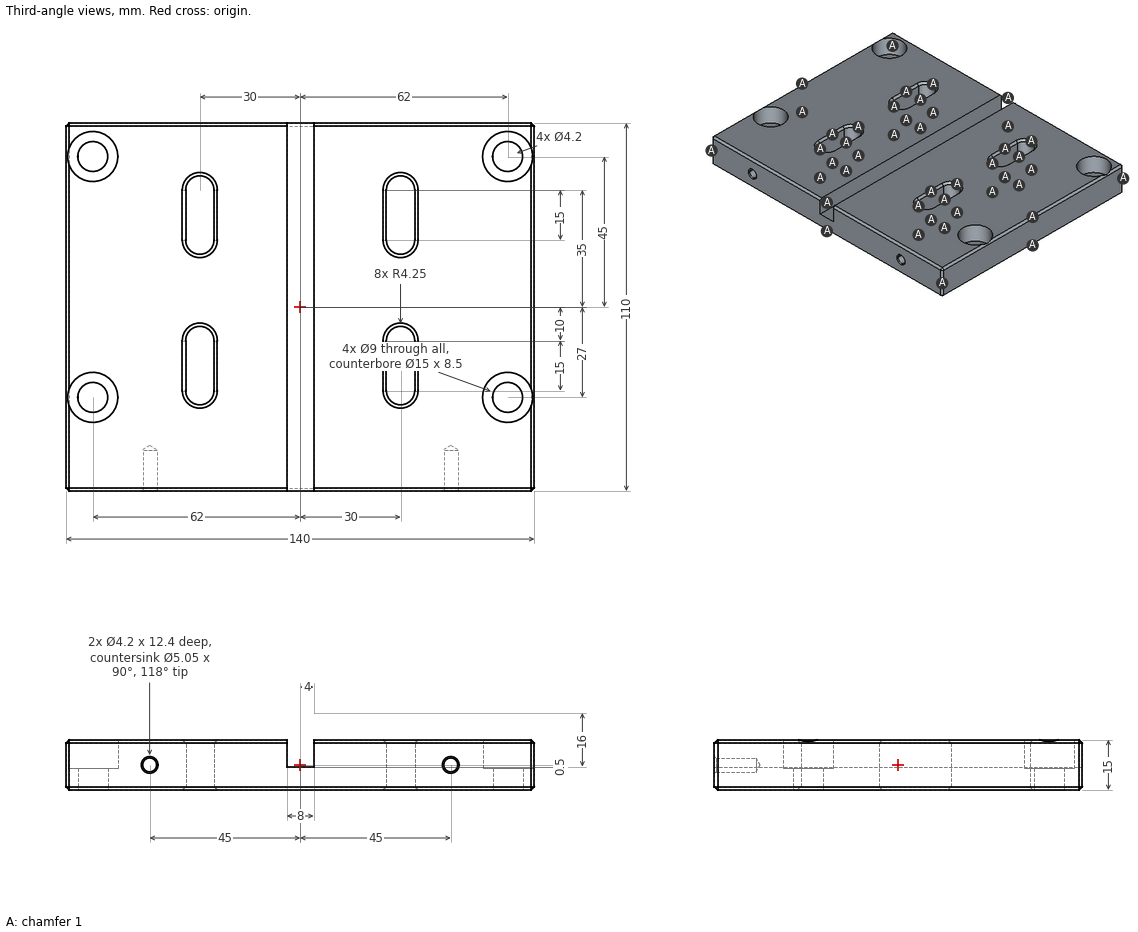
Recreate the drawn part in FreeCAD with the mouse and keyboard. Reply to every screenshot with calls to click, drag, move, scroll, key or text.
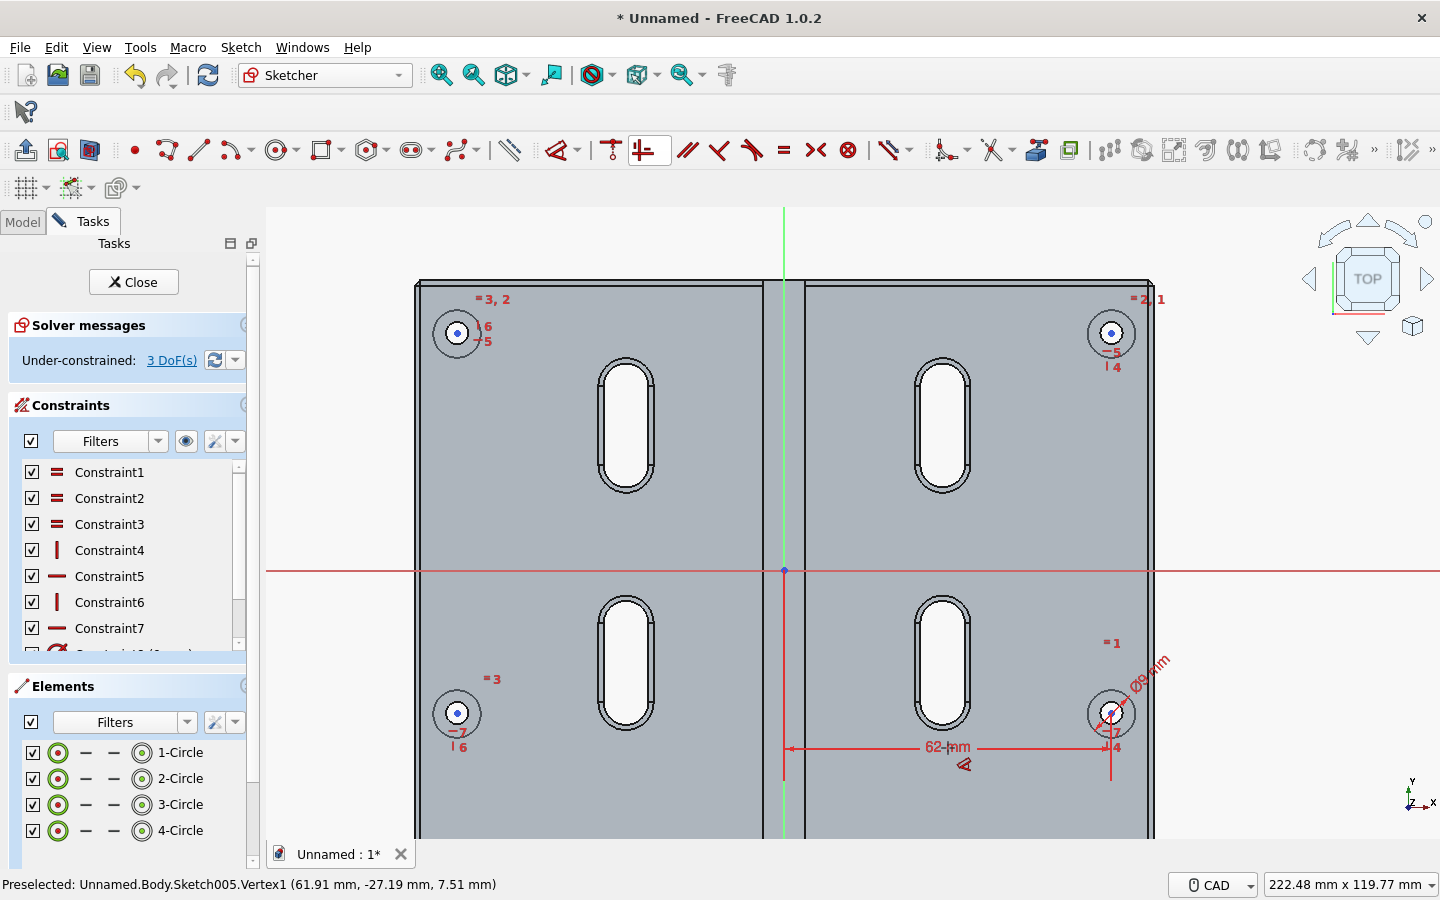
click(1111, 714)
click(1145, 642)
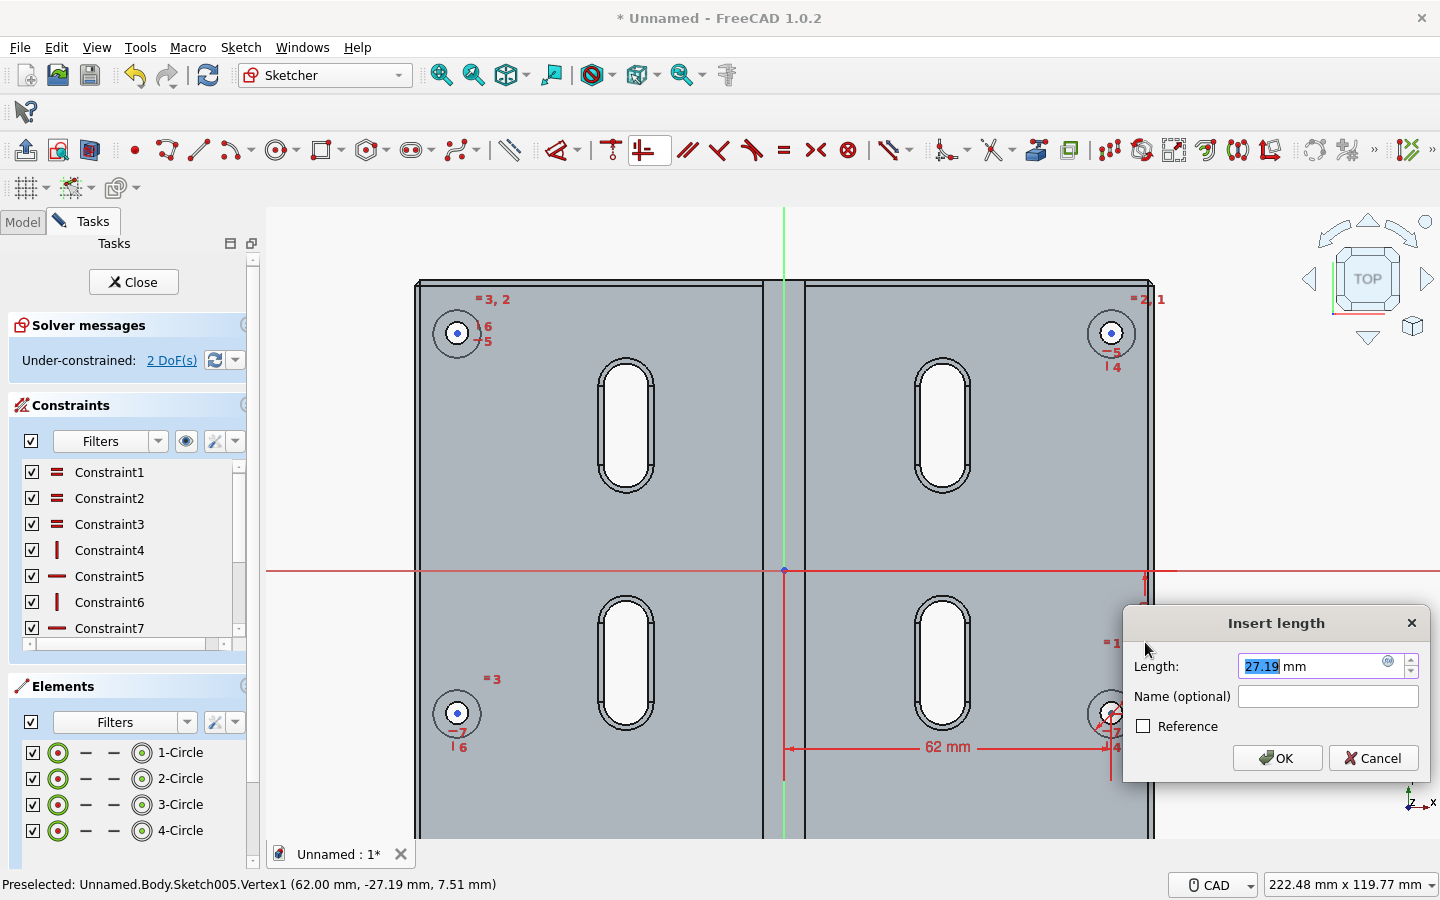
text(27)
key(Return)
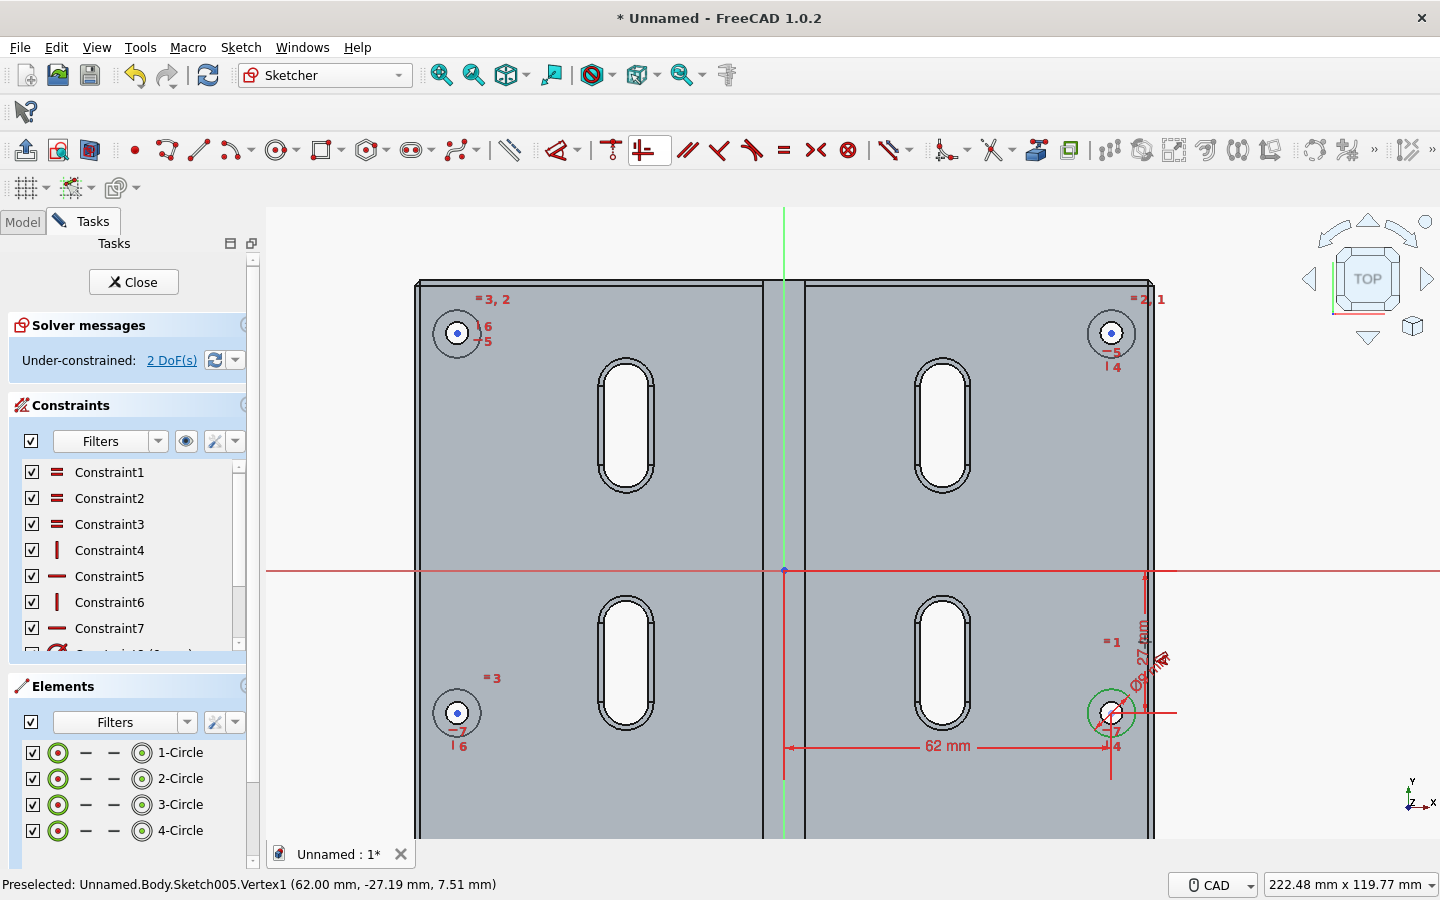
click(1111, 334)
click(1145, 452)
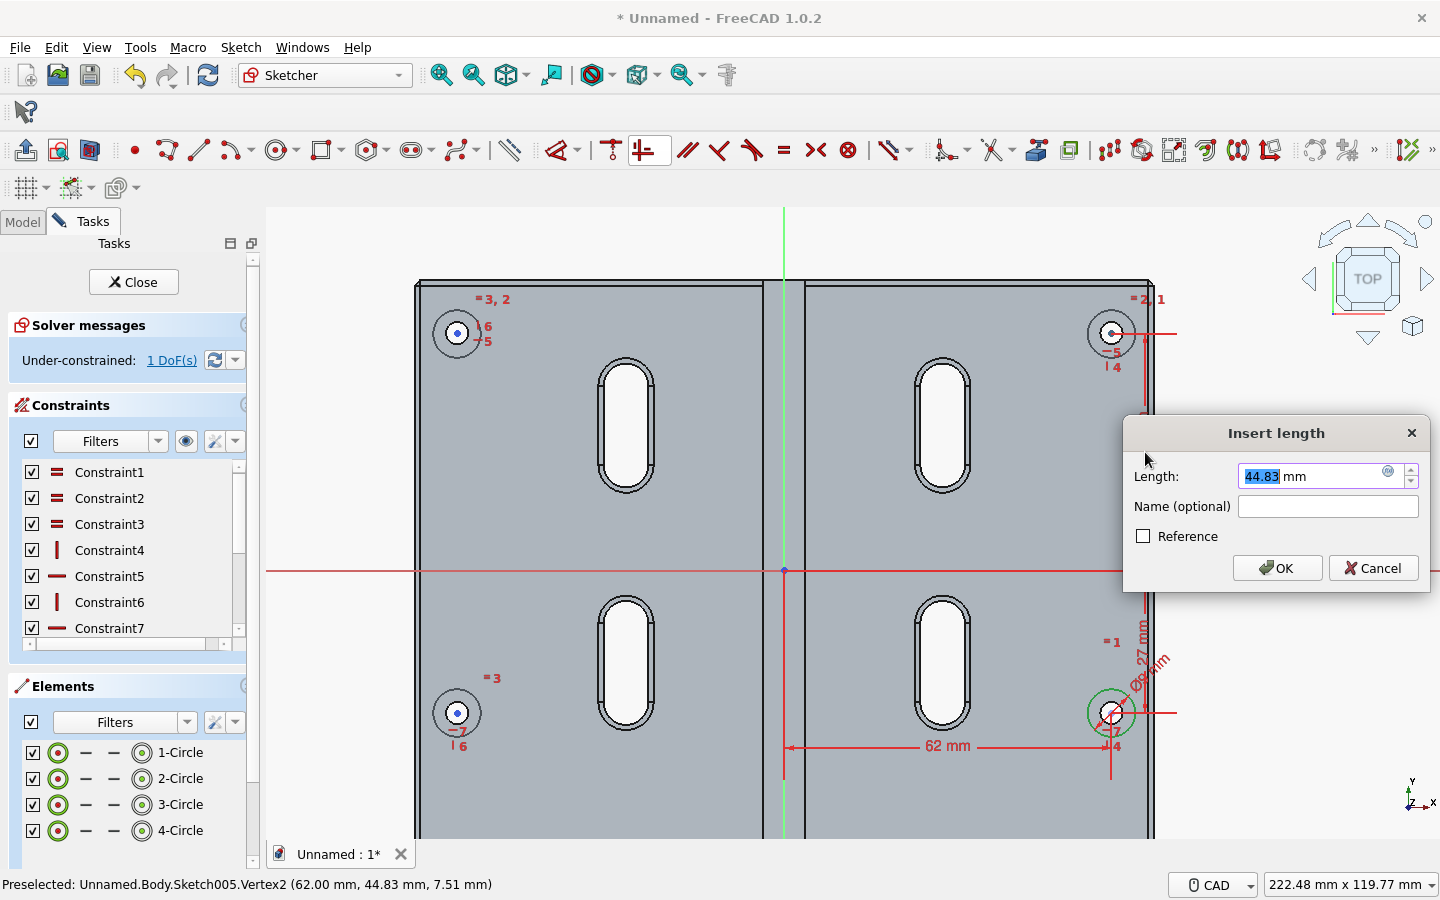
text(45)
key(Return)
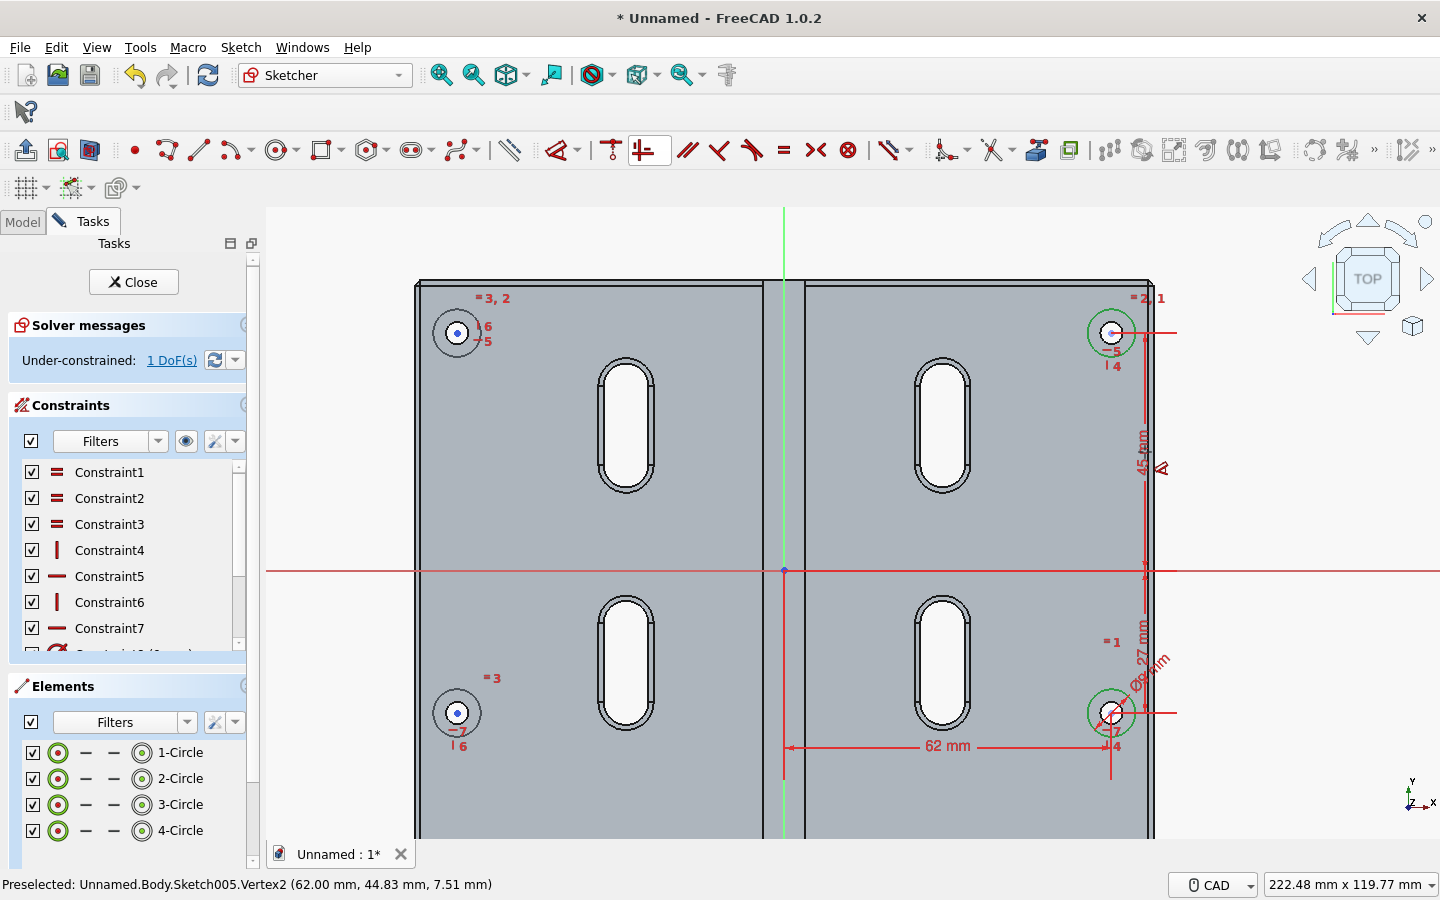
click(457, 333)
click(621, 299)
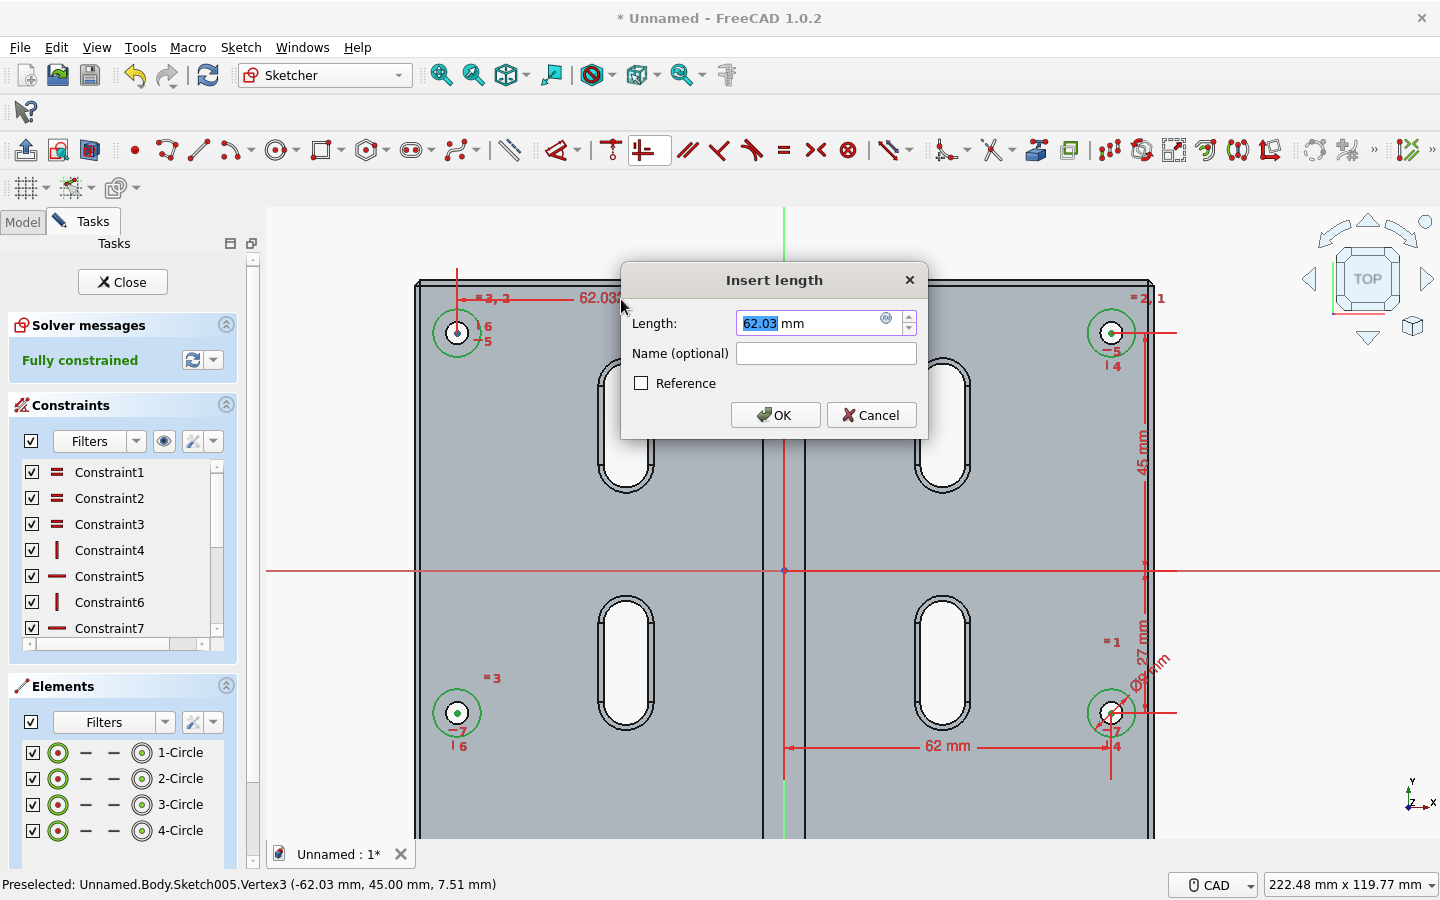
text(62)
key(Return)
key(Escape)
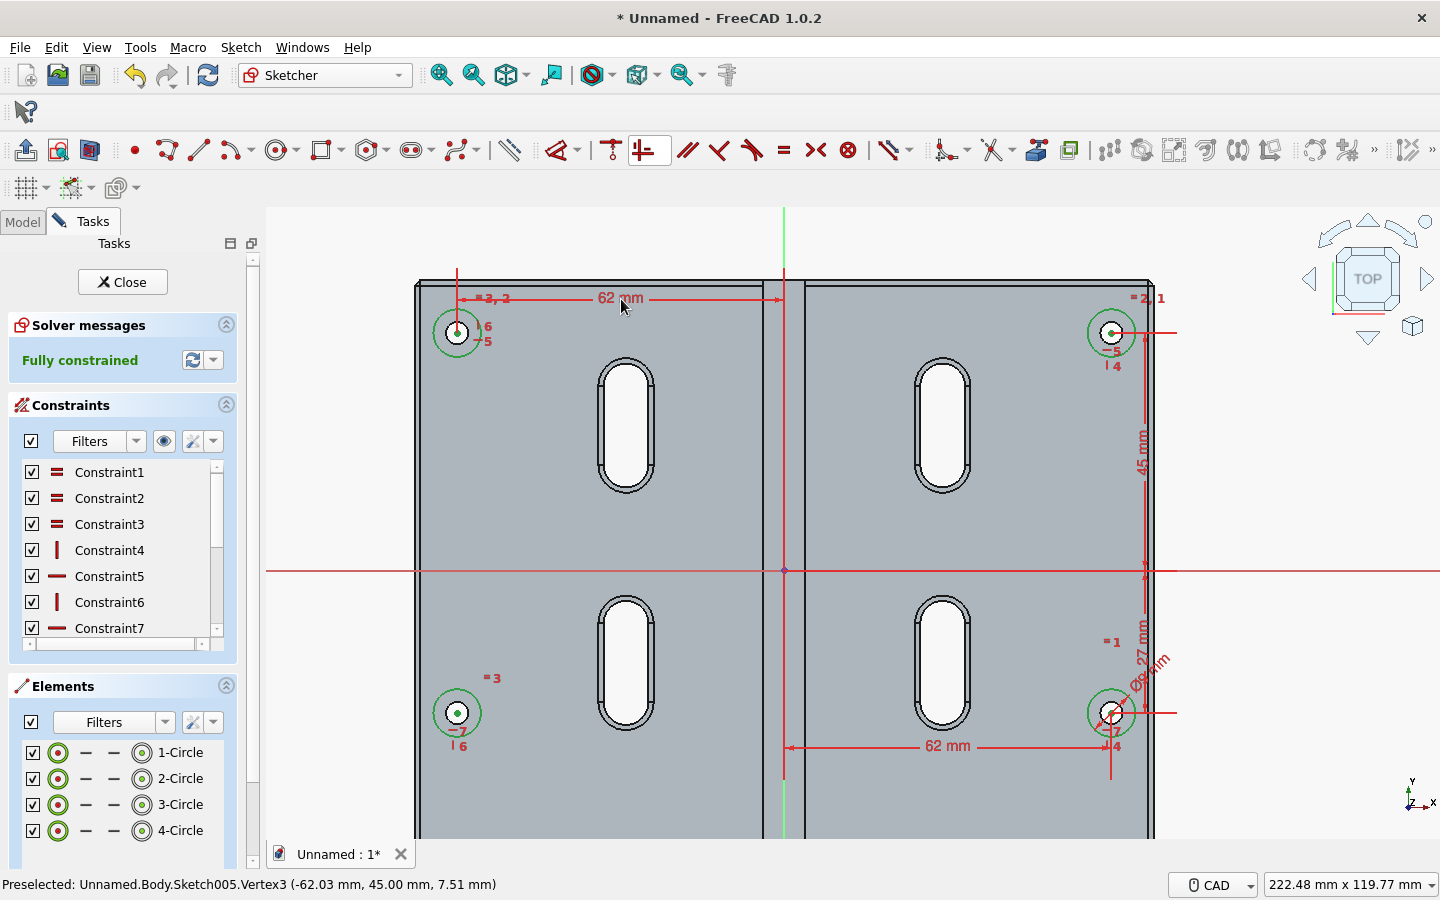
click(123, 282)